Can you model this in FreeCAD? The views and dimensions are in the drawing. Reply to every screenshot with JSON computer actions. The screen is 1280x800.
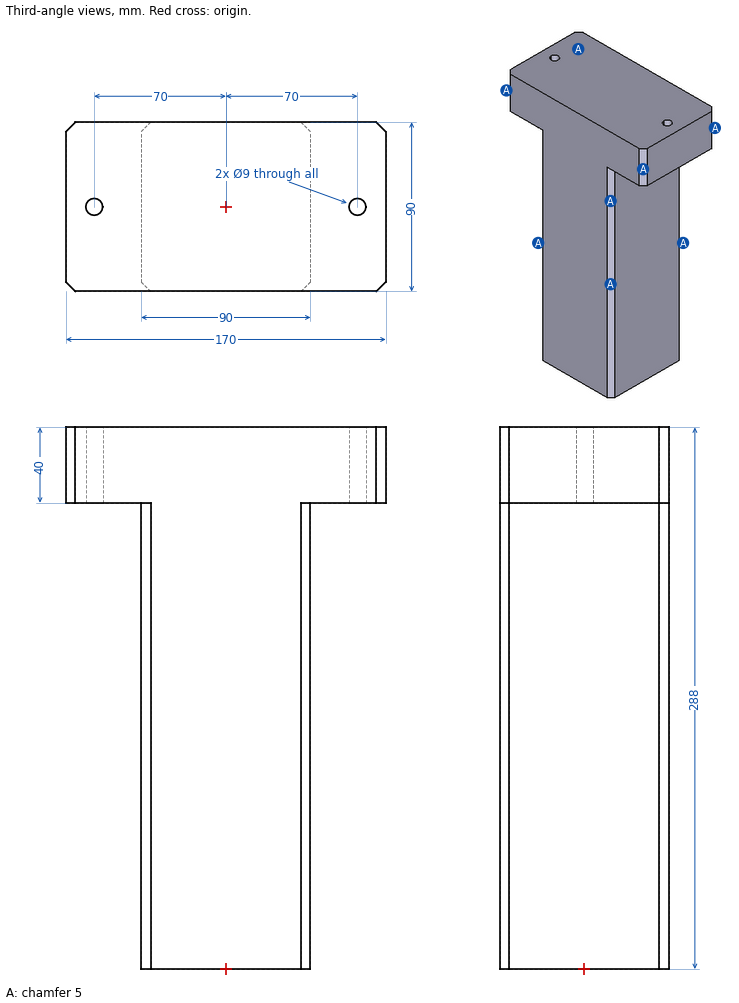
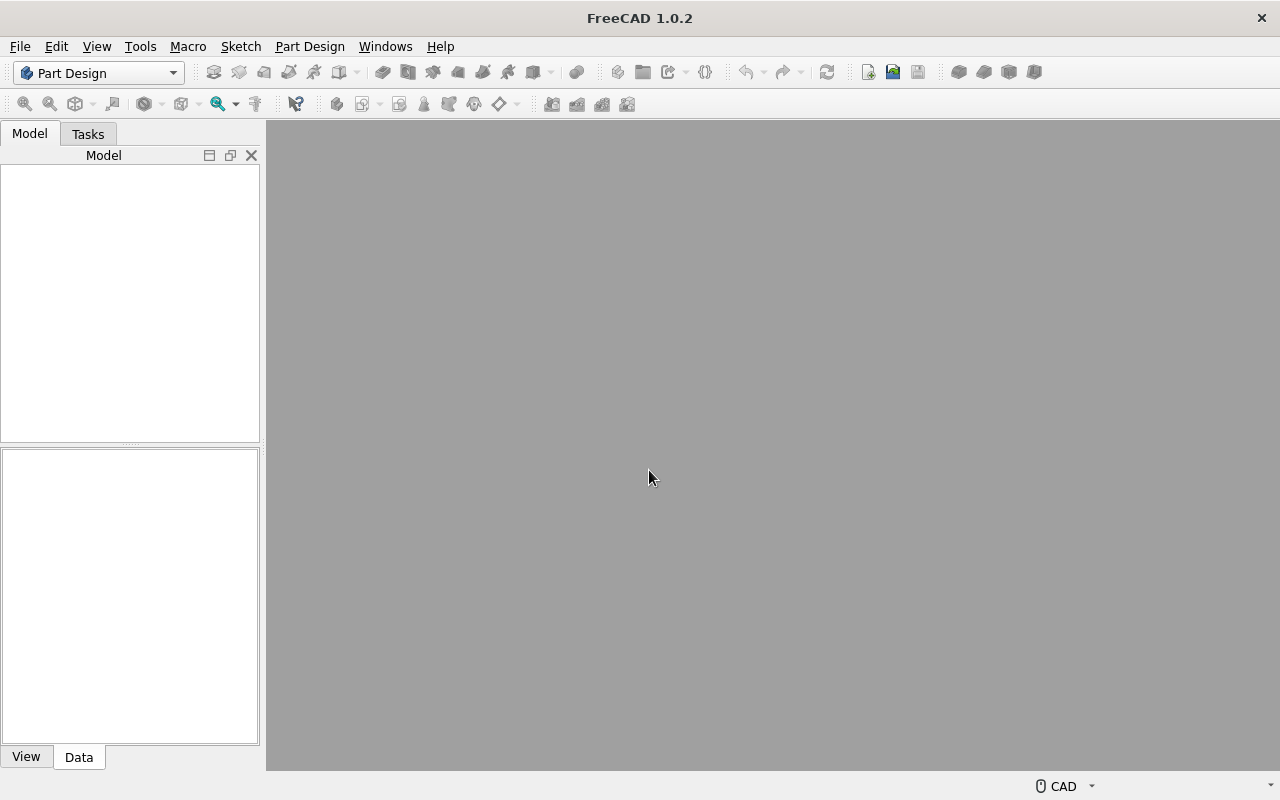
{"action": "left_click", "coordinate": [868, 72]}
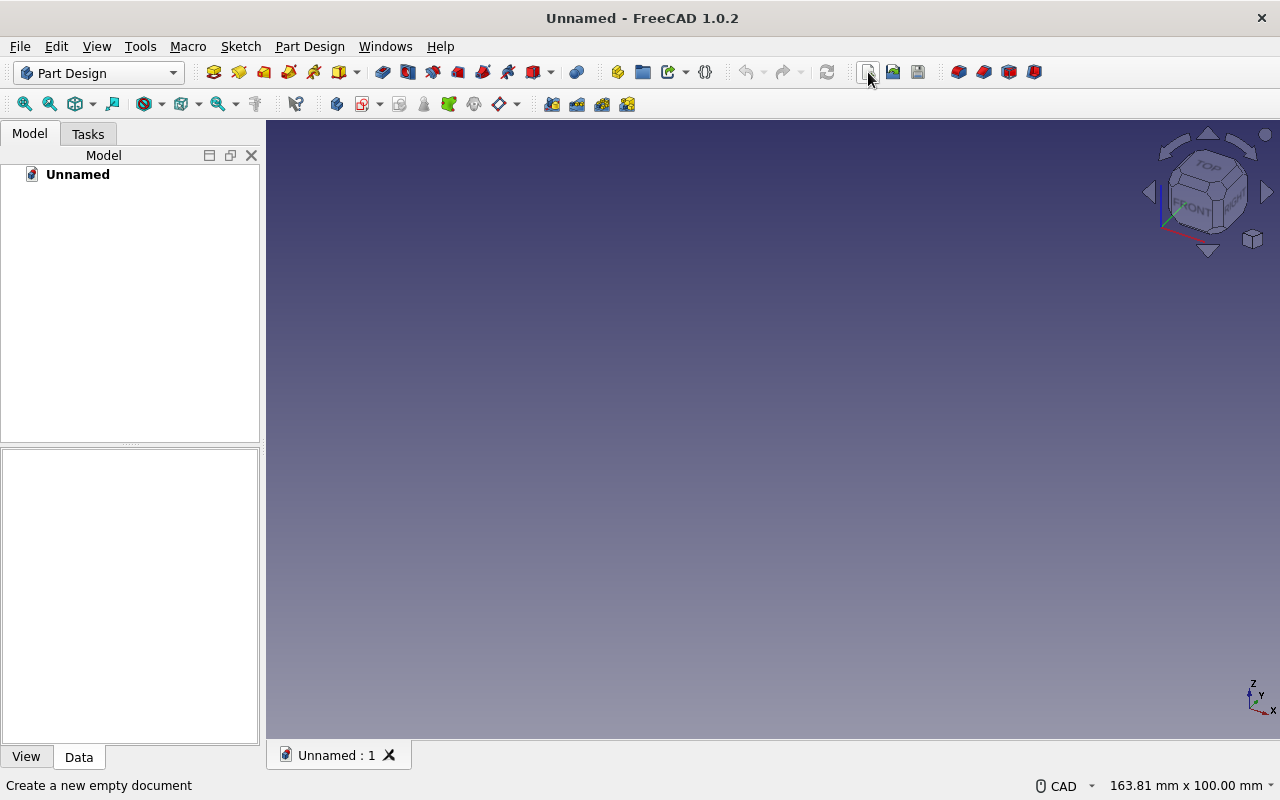
{"action": "left_click", "coordinate": [362, 104]}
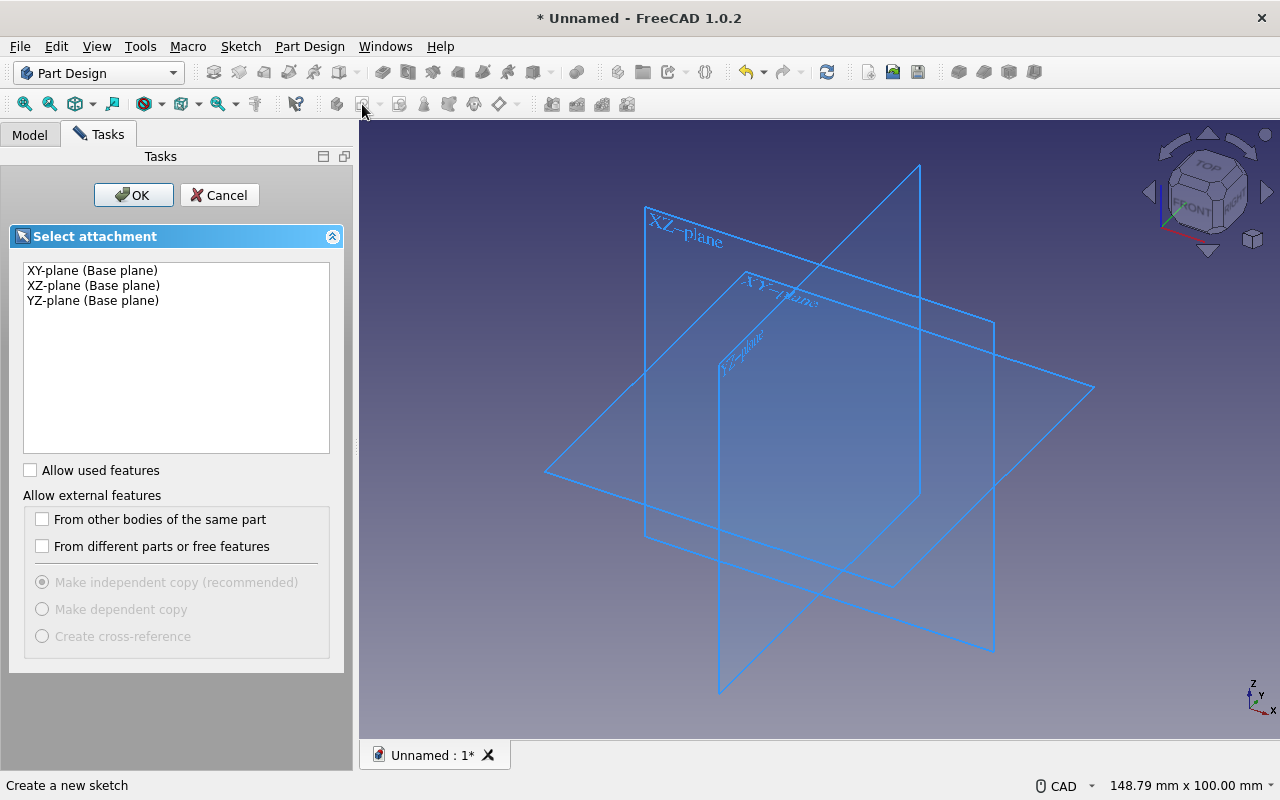
{"action": "left_click", "coordinate": [84, 270]}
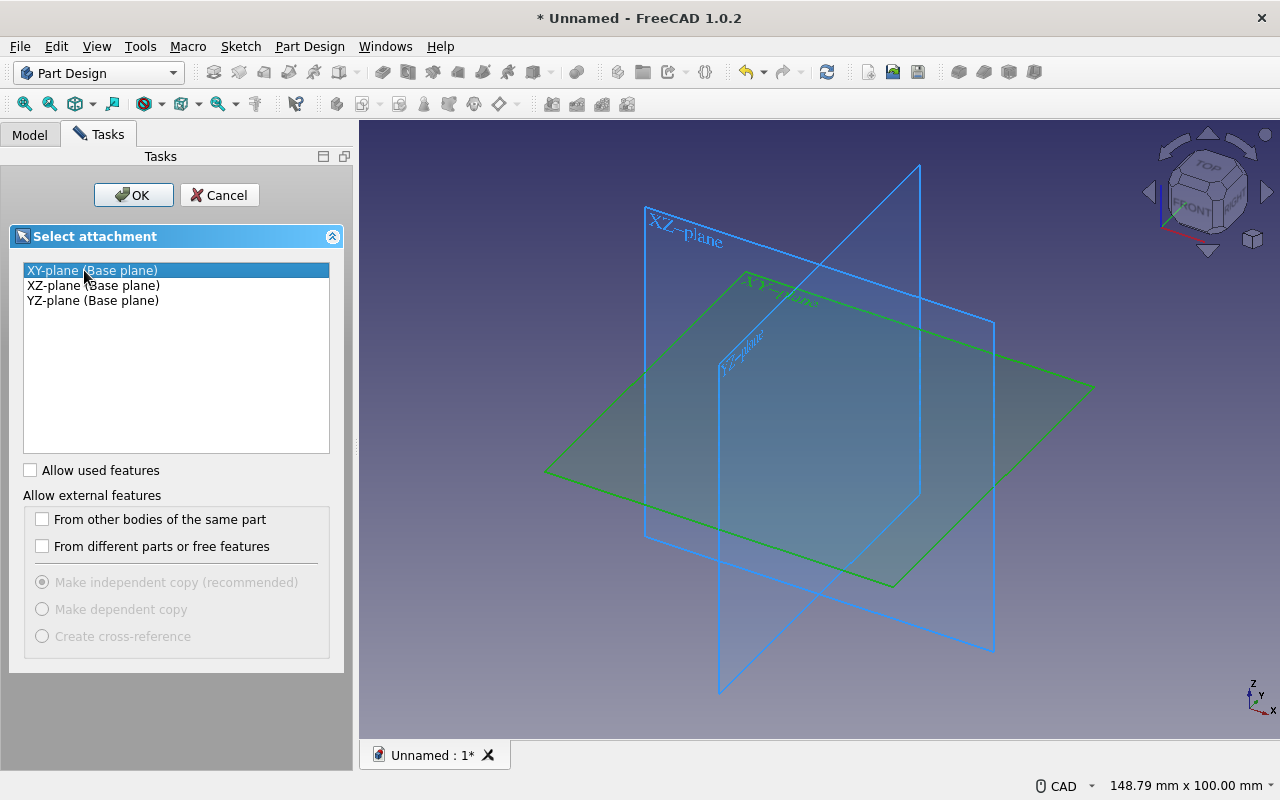
{"action": "left_click", "coordinate": [134, 195]}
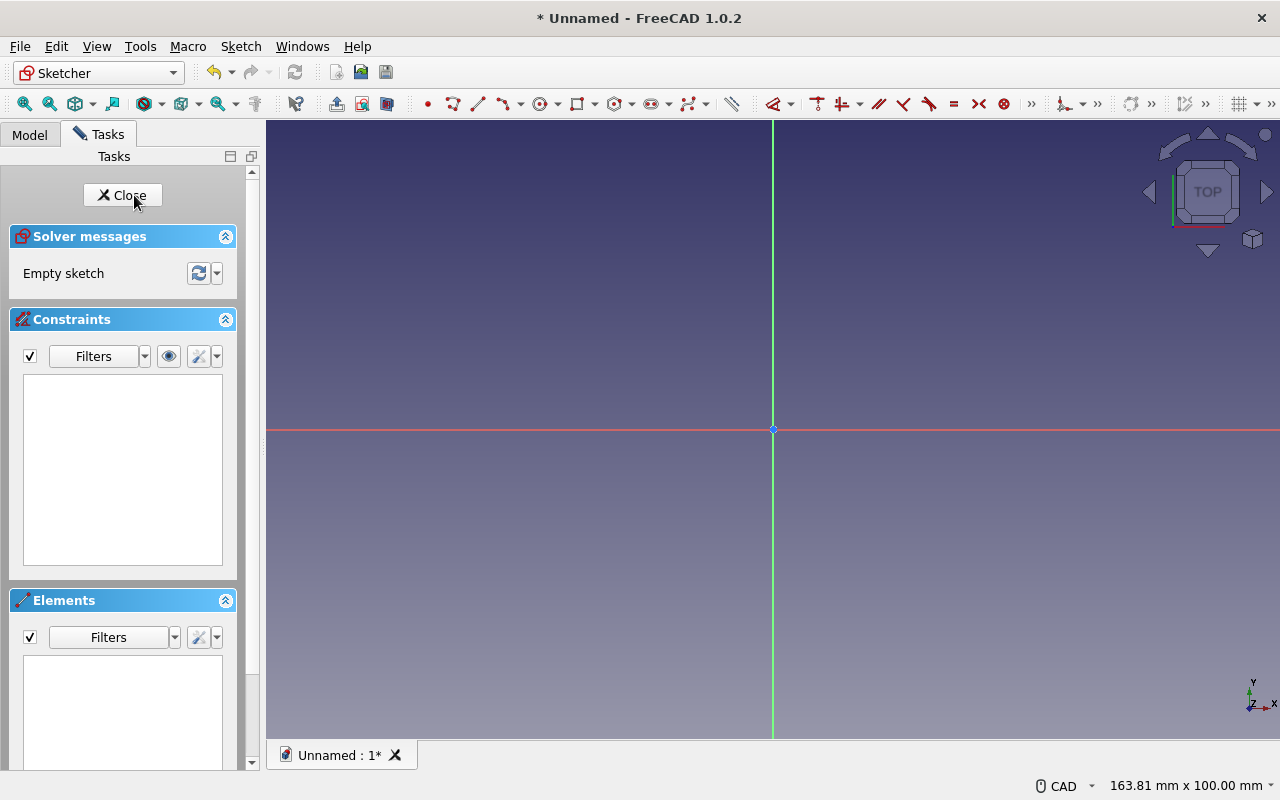
{"action": "scroll", "coordinate": [565, 429], "scroll_direction": "down", "scroll_amount": 2}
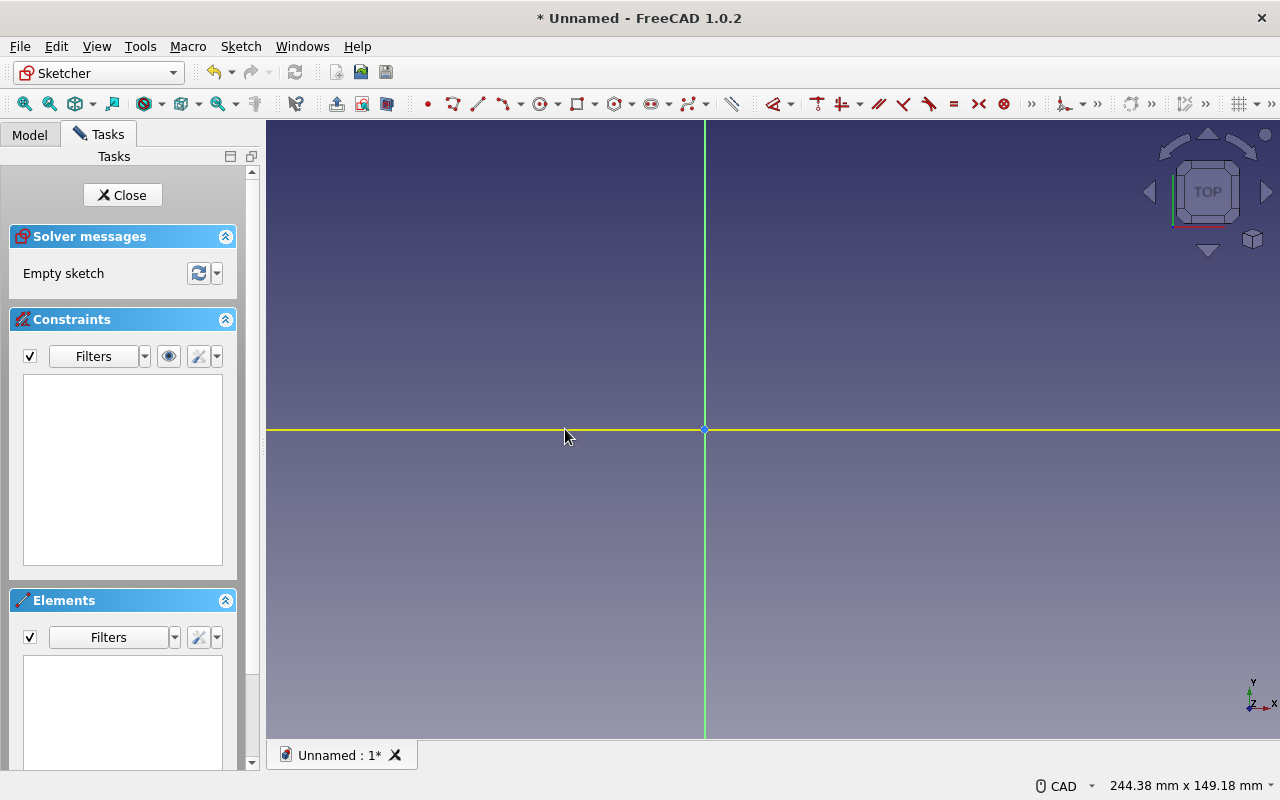
{"action": "left_click", "coordinate": [594, 104]}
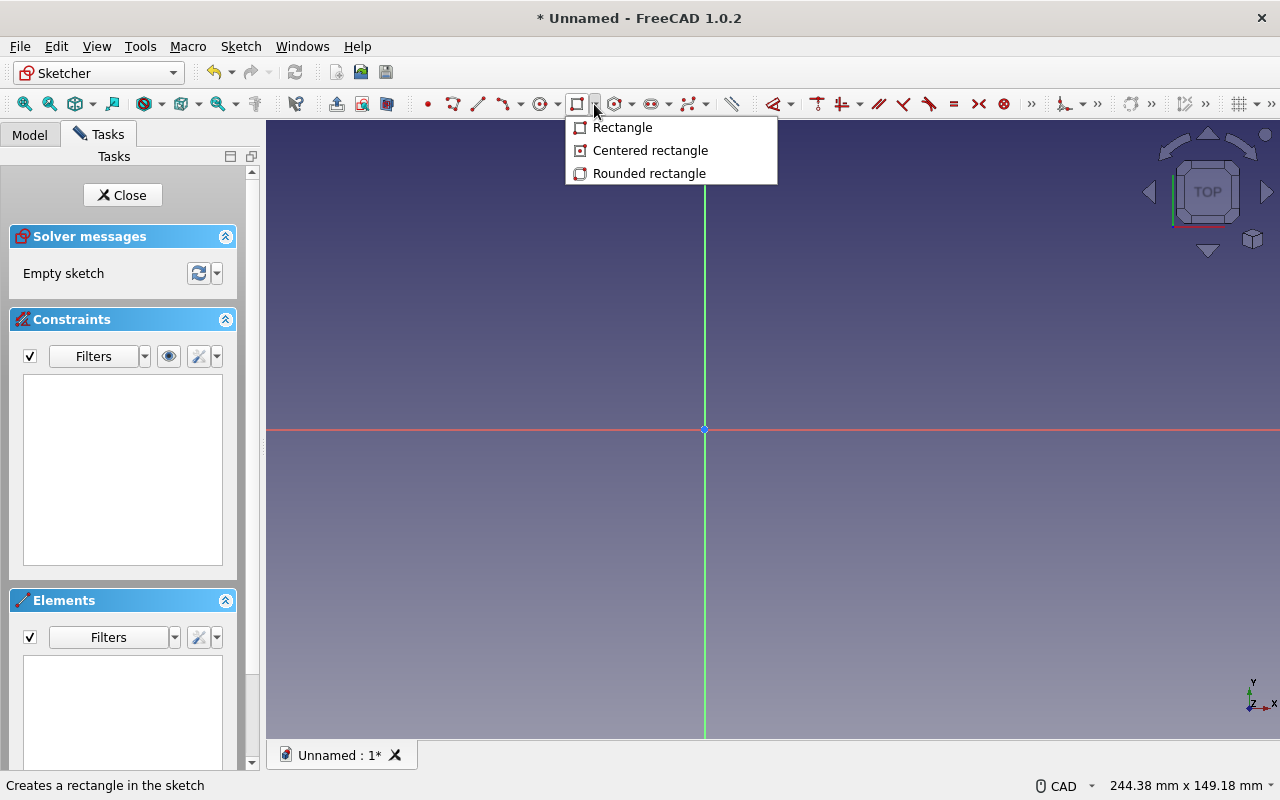
{"action": "left_click", "coordinate": [672, 150]}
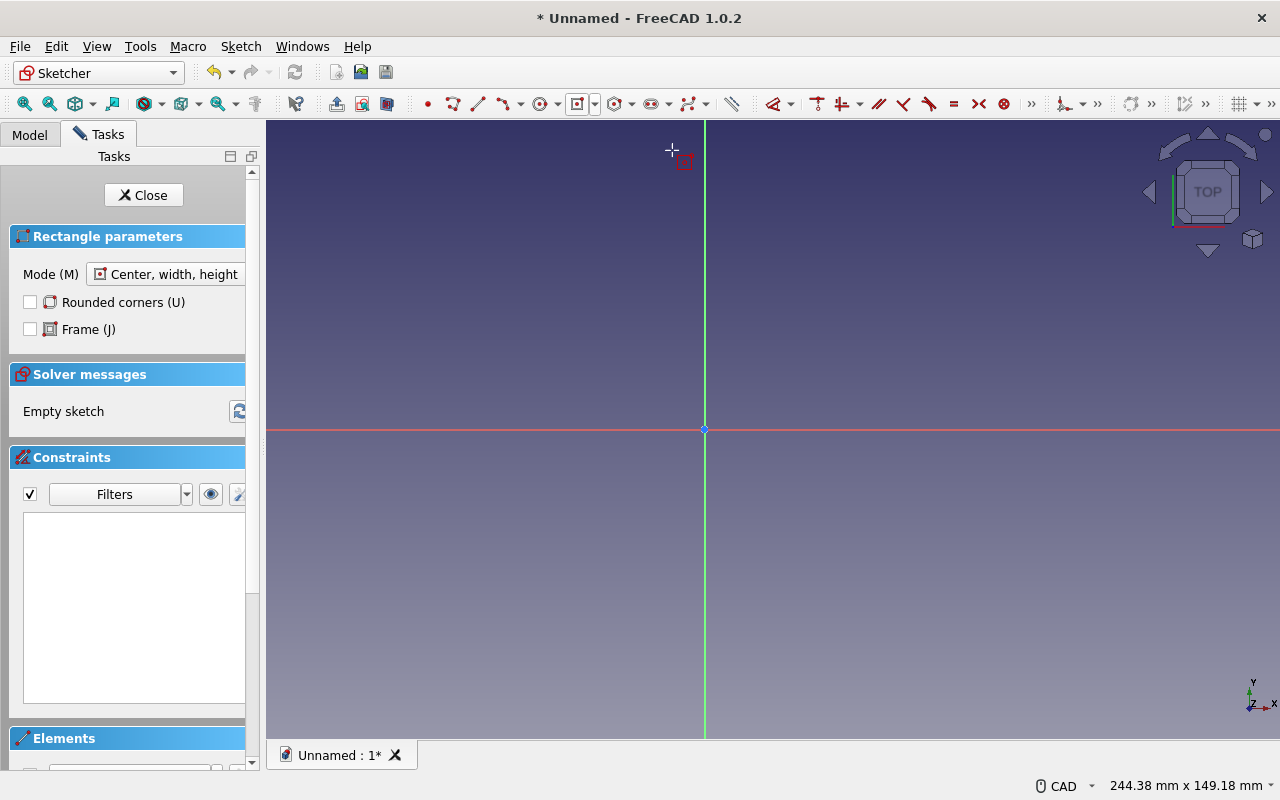
{"action": "left_click", "coordinate": [705, 430]}
{"action": "left_click", "coordinate": [891, 243]}
{"action": "key", "text": "Escape"}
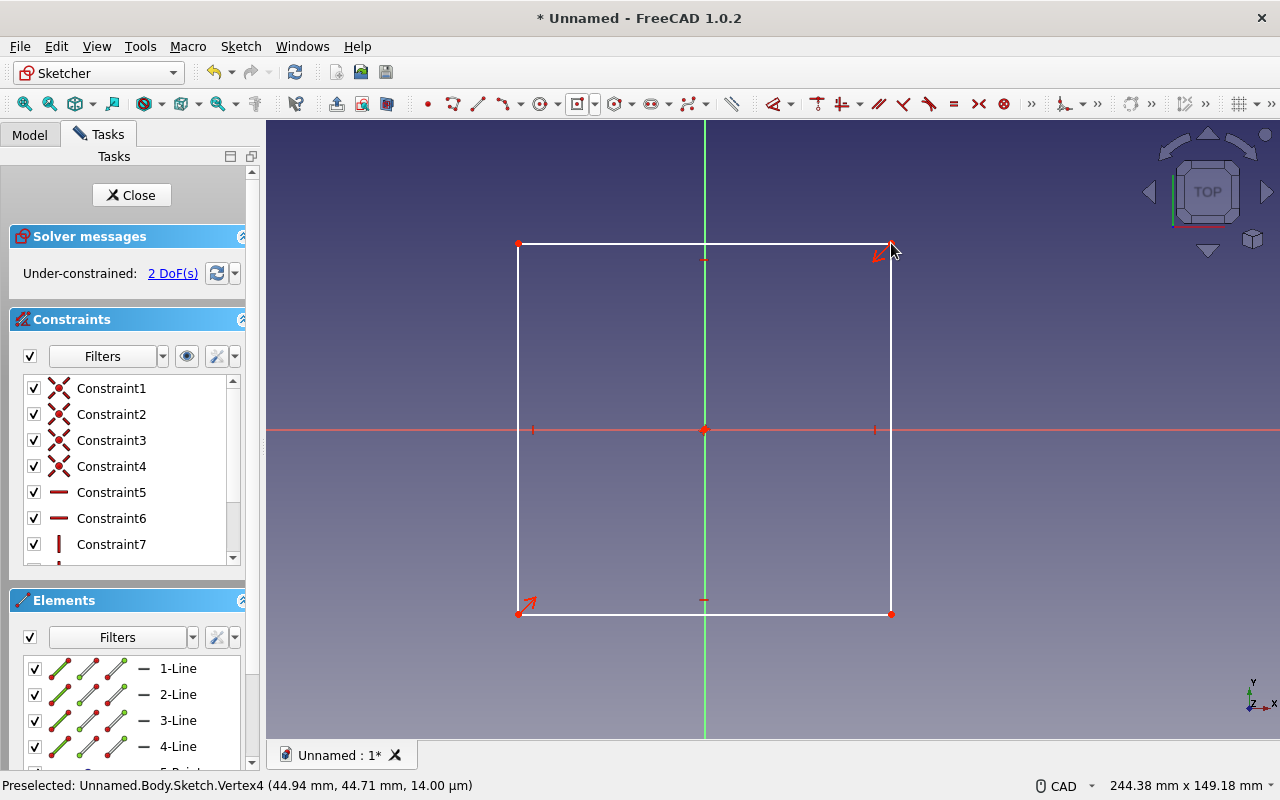
{"action": "left_click", "coordinate": [630, 615]}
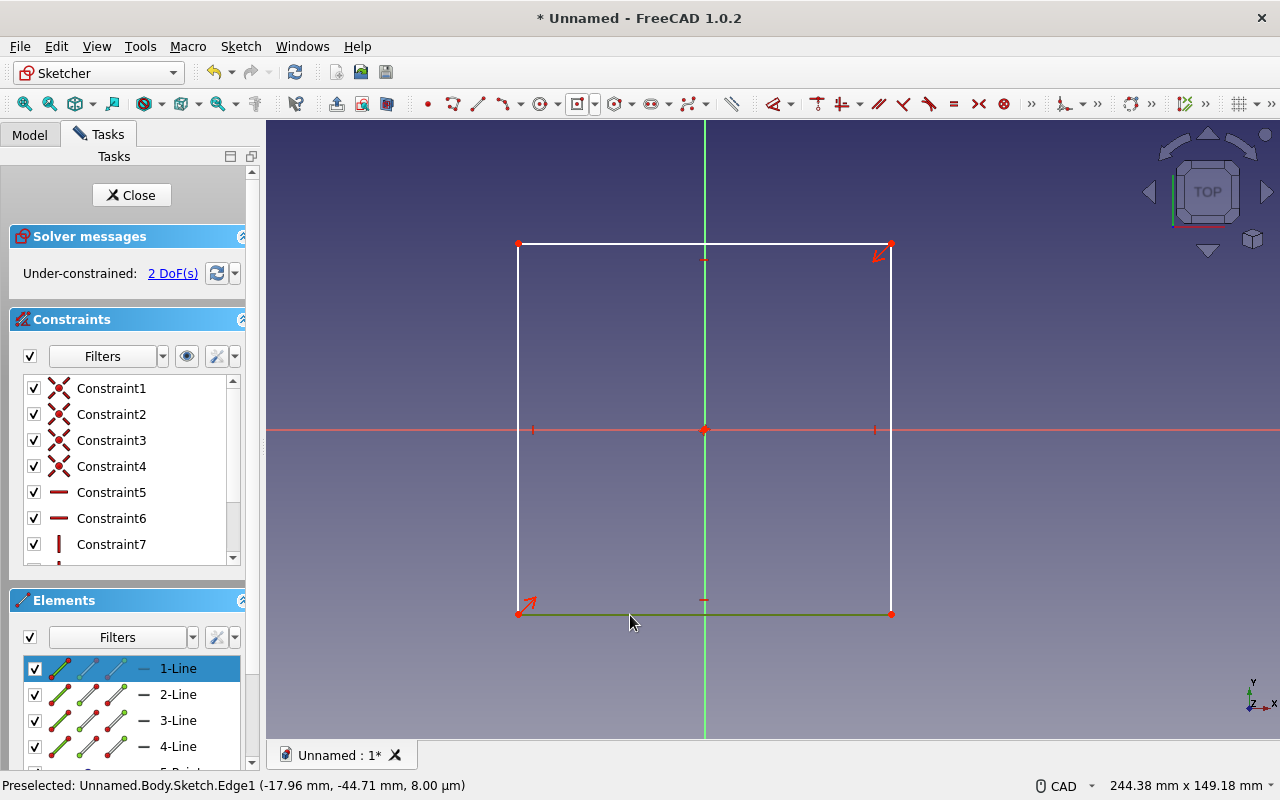
{"action": "key", "text": "l"}